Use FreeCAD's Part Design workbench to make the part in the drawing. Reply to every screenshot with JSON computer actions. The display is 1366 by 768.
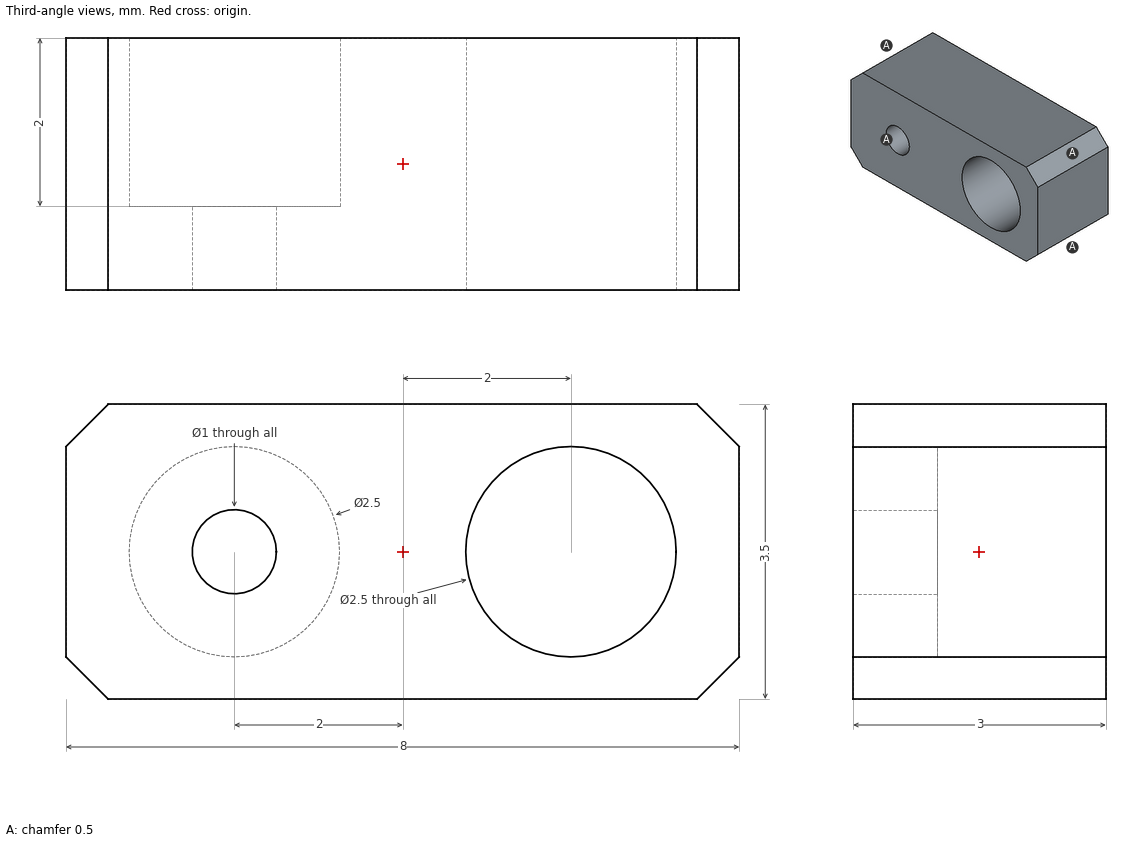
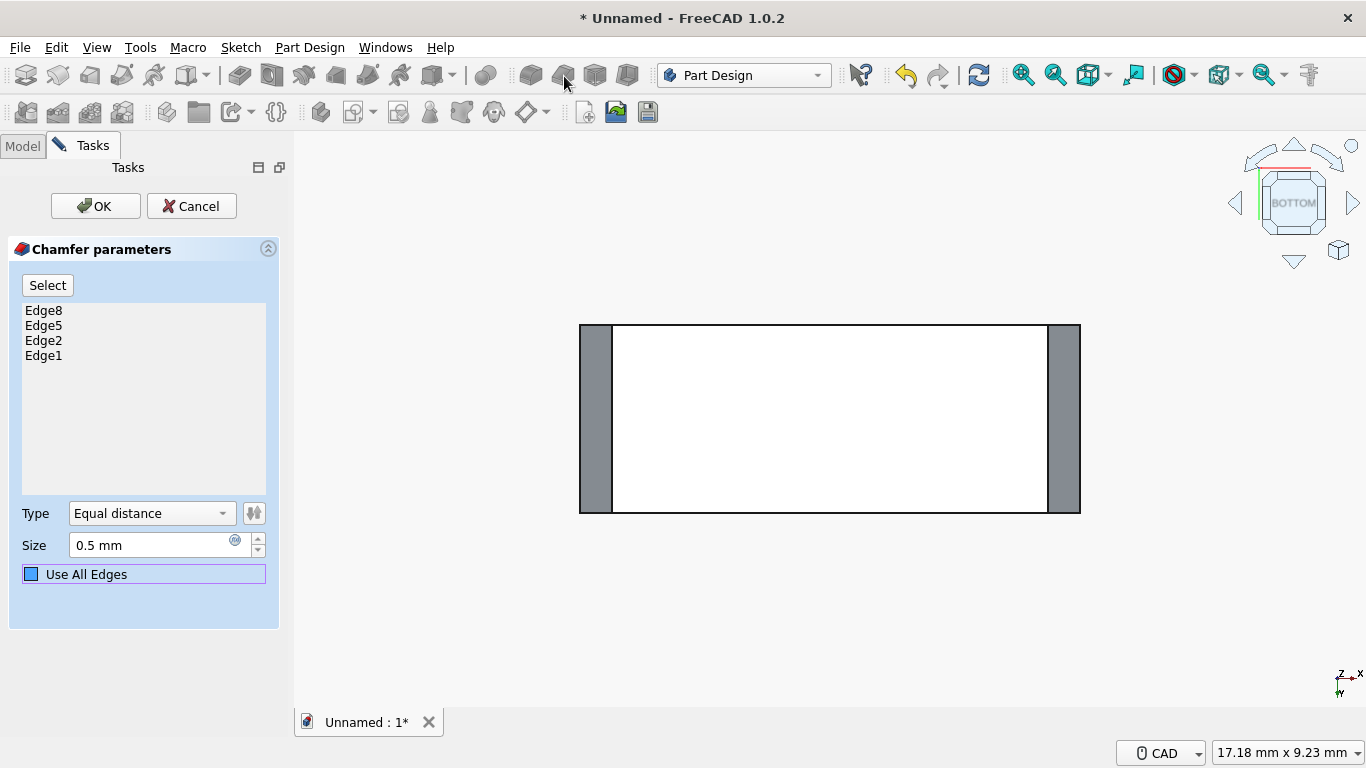
{"action": "left_click", "coordinate": [96, 206]}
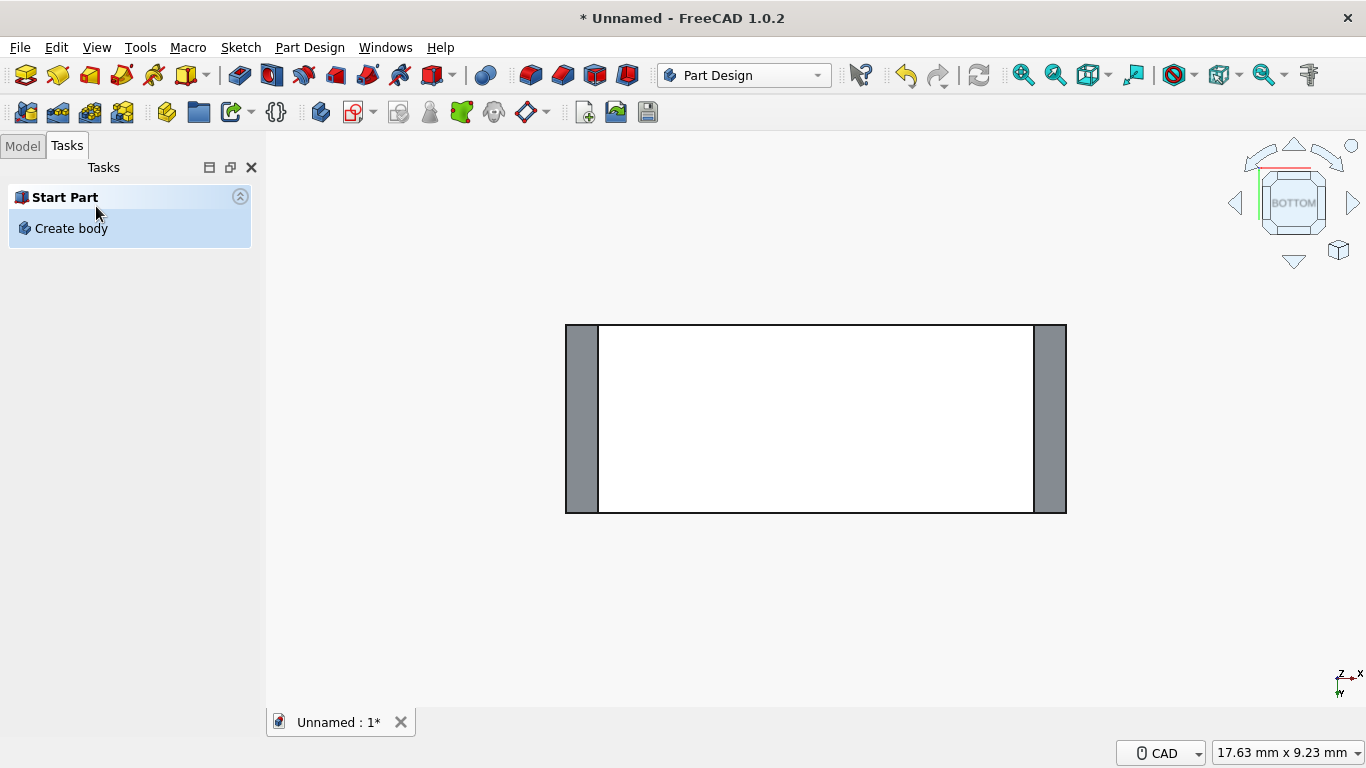
{"action": "key", "text": "0"}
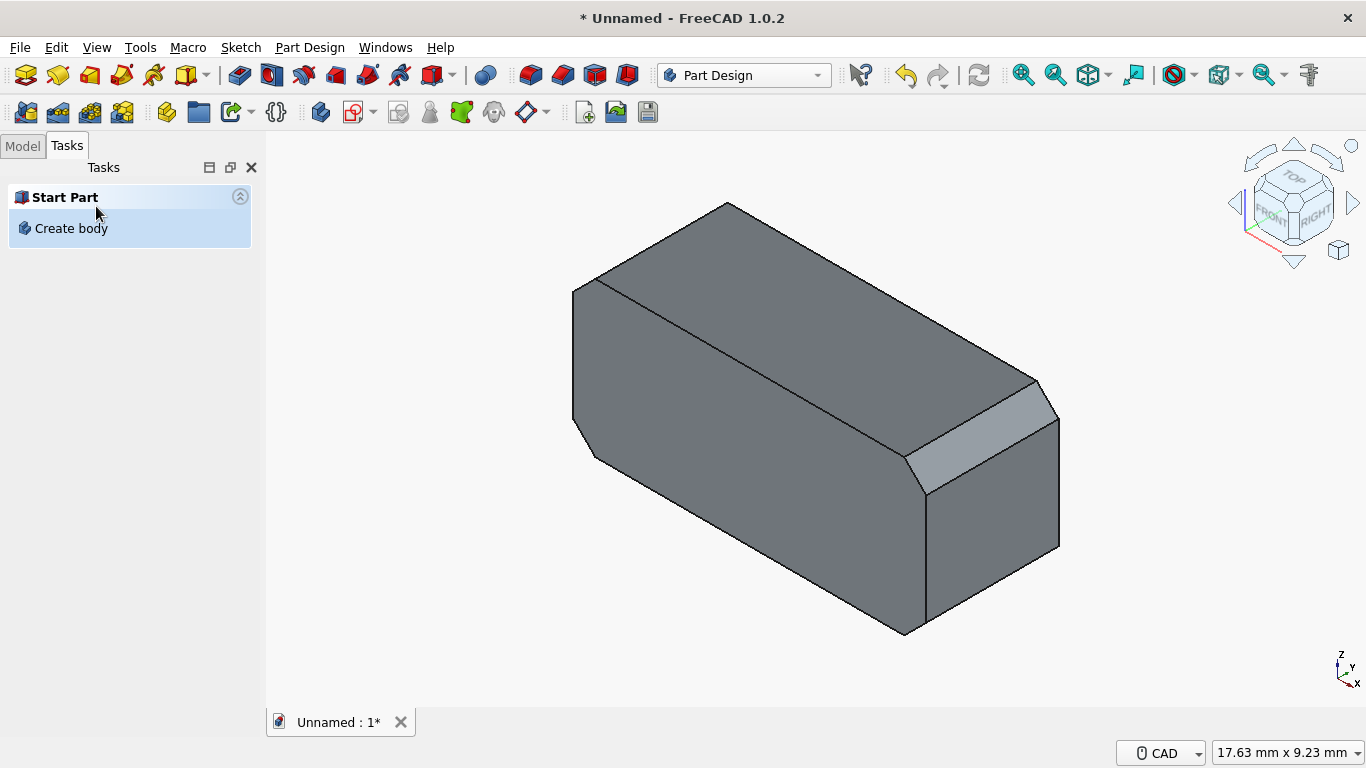
{"action": "left_click", "coordinate": [800, 485]}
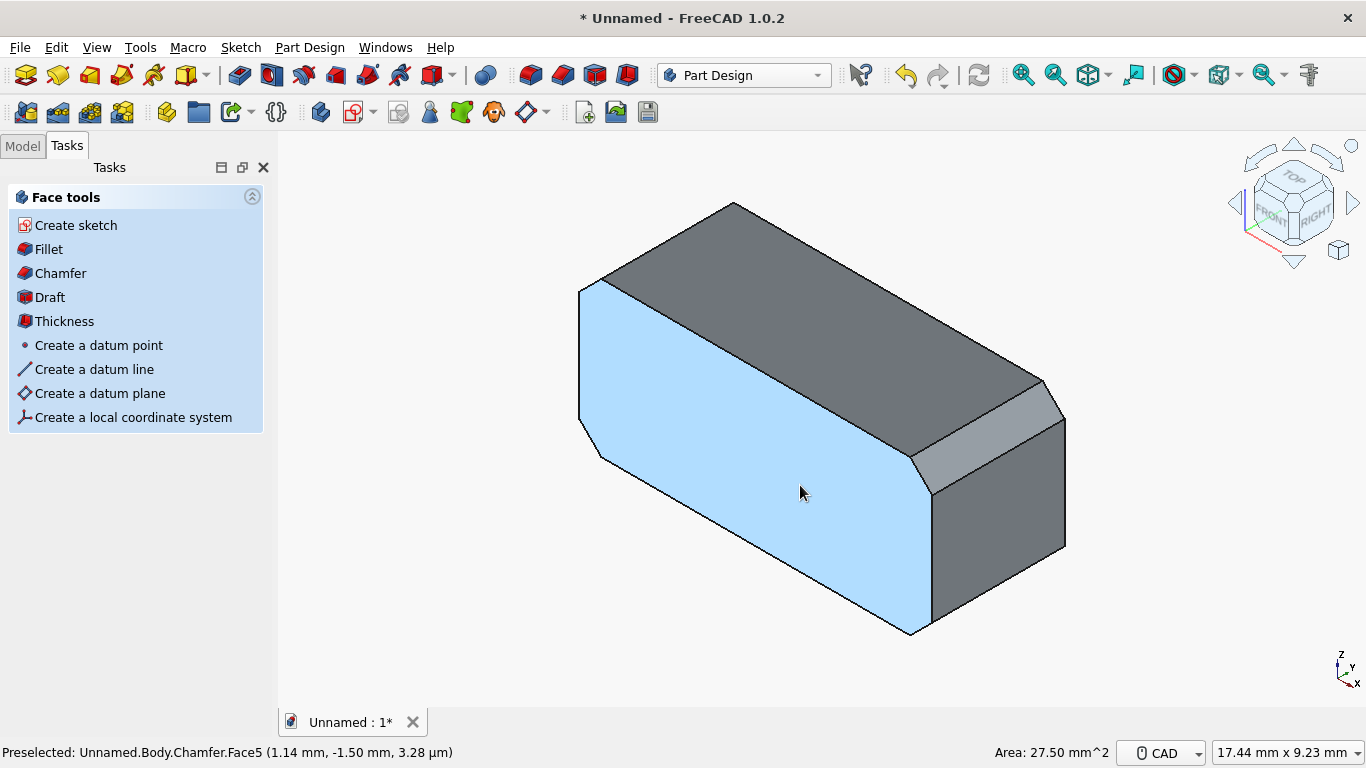
{"action": "left_click", "coordinate": [354, 112]}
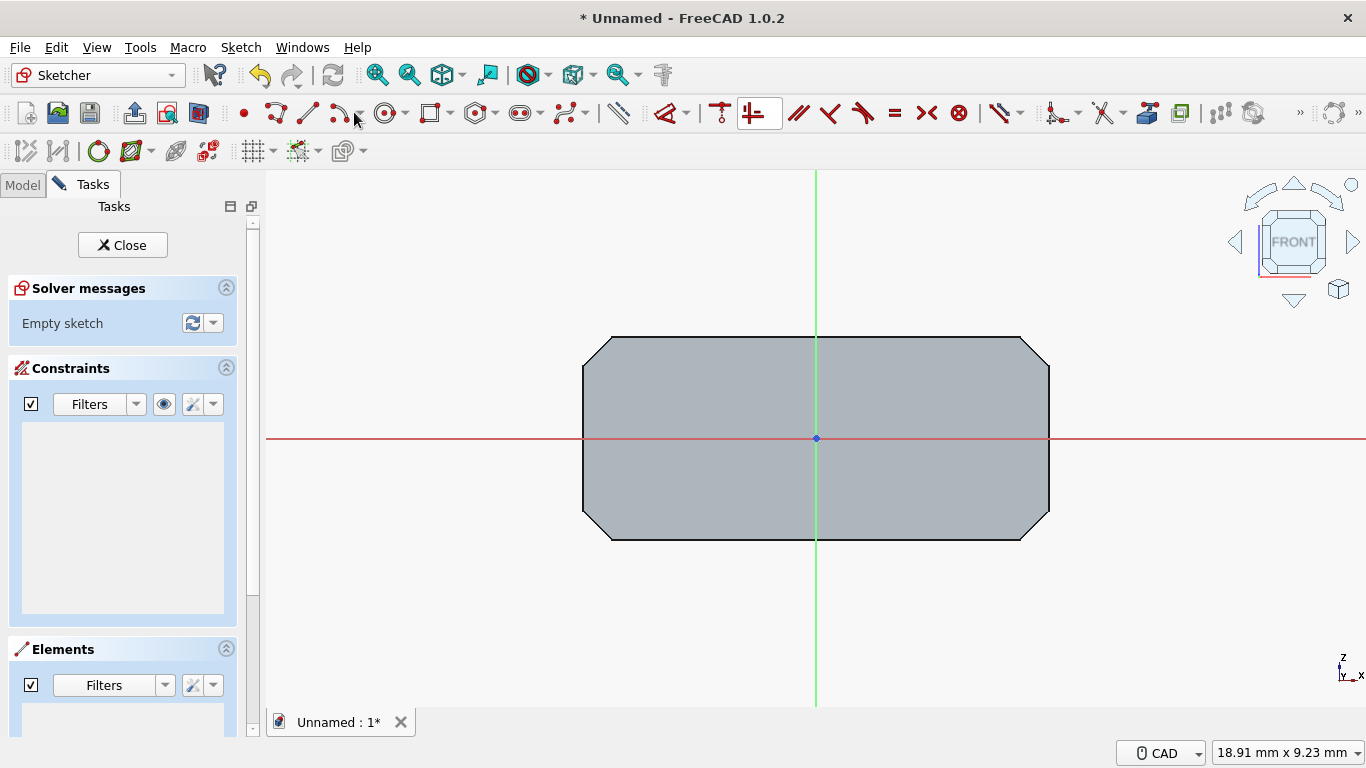
{"action": "scroll", "coordinate": [690, 438], "scroll_direction": "up", "scroll_amount": 9}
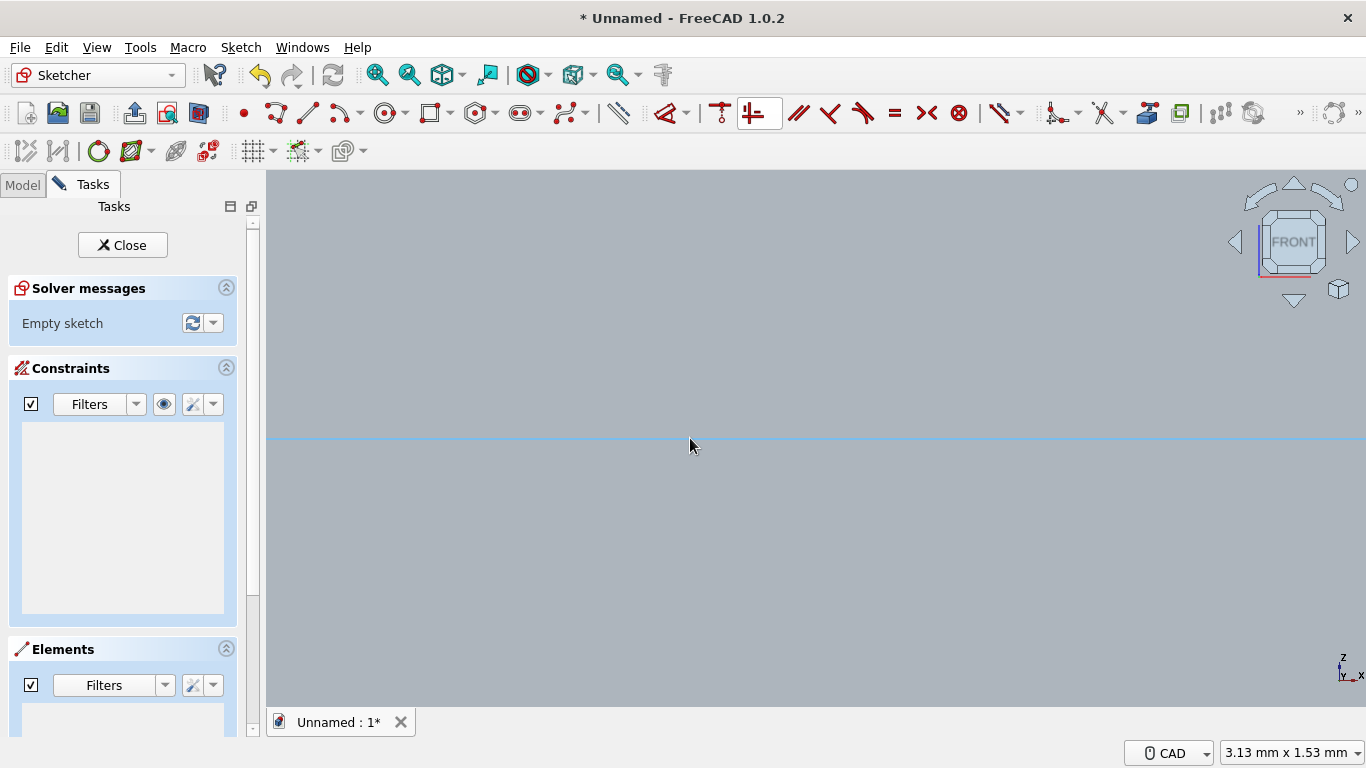
{"action": "left_click", "coordinate": [386, 114]}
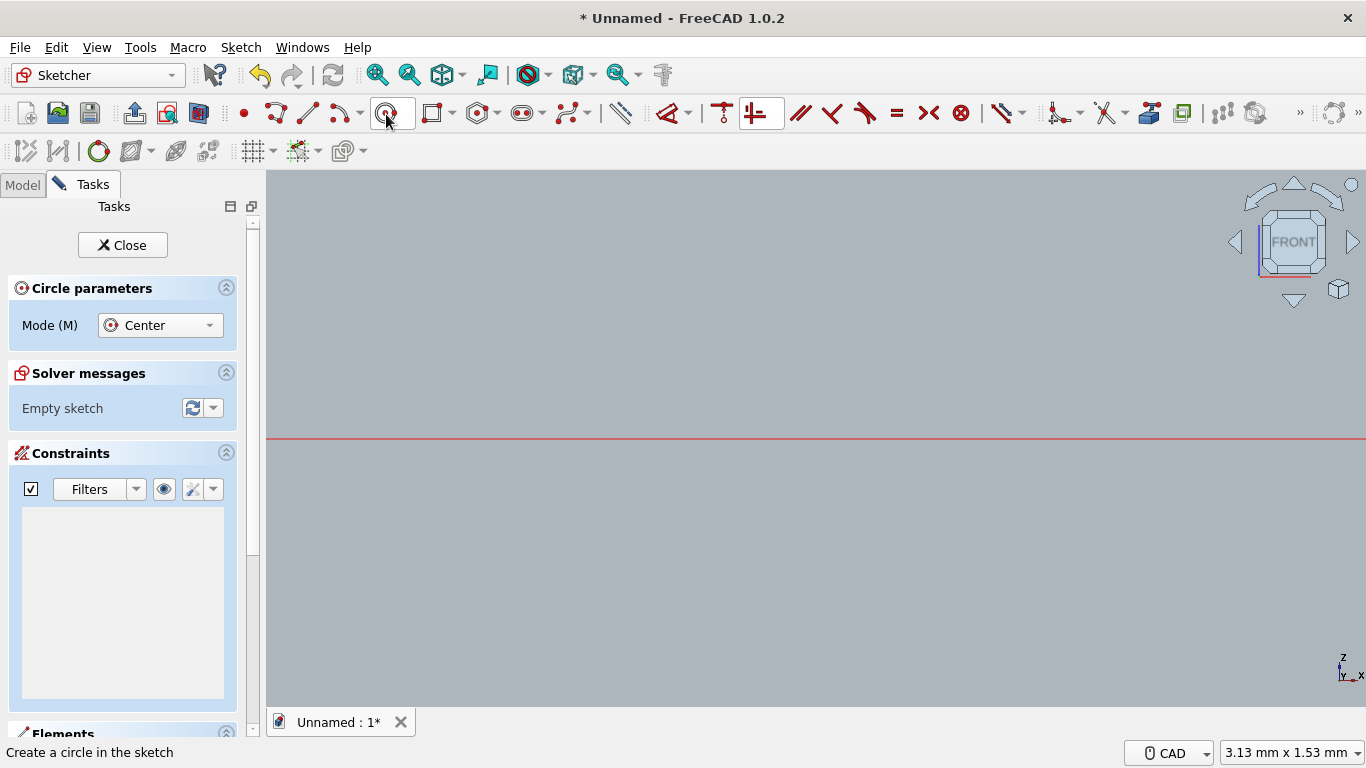
{"action": "left_click", "coordinate": [747, 438]}
{"action": "left_click", "coordinate": [871, 314]}
{"action": "key", "text": "Escape"}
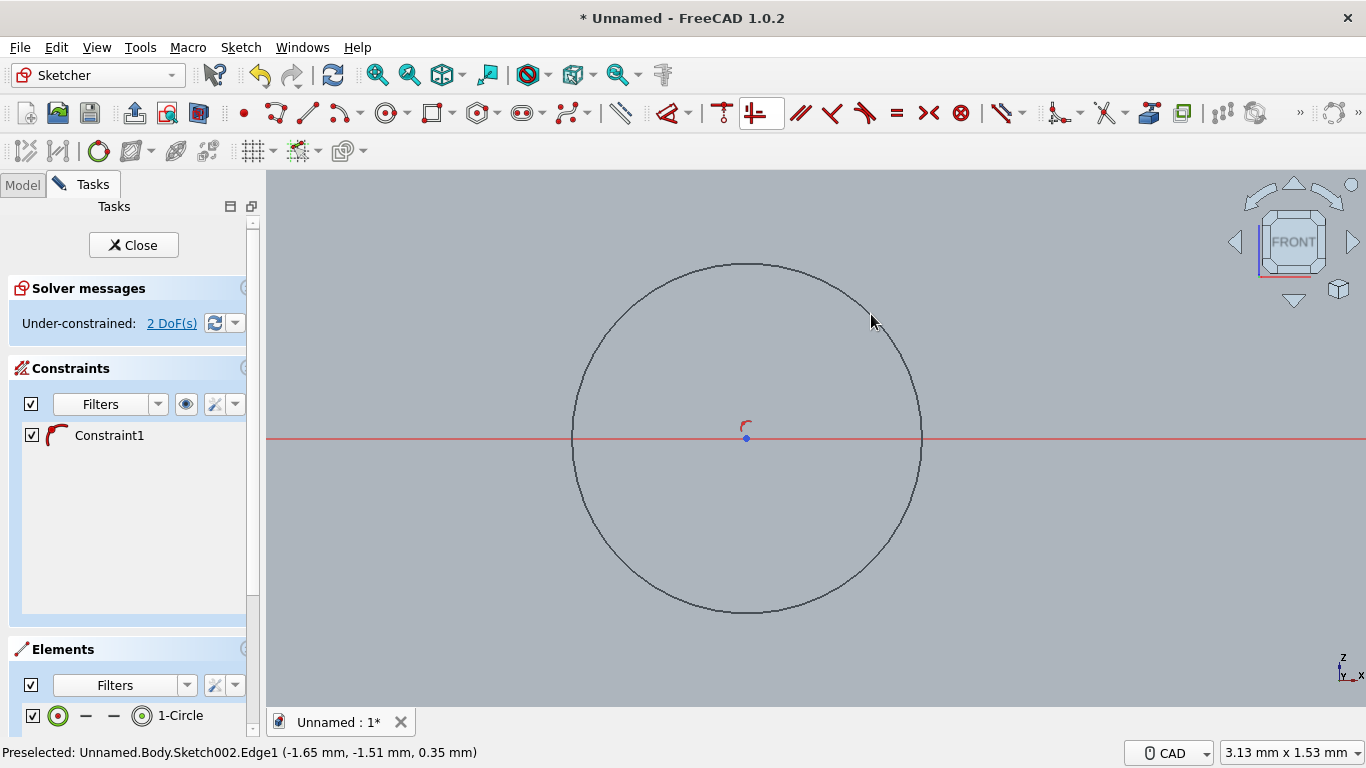
{"action": "left_click", "coordinate": [668, 114]}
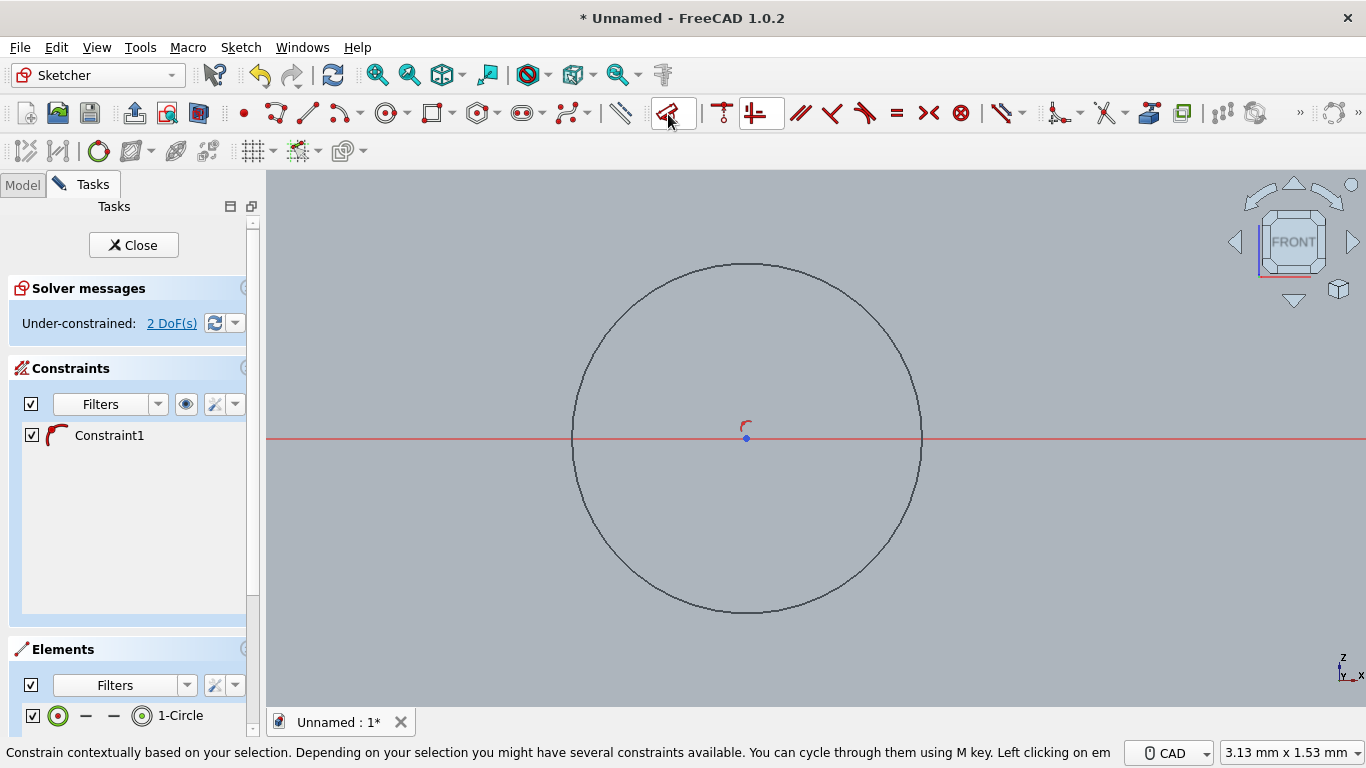
{"action": "left_click", "coordinate": [870, 314]}
{"action": "left_click", "coordinate": [892, 291]}